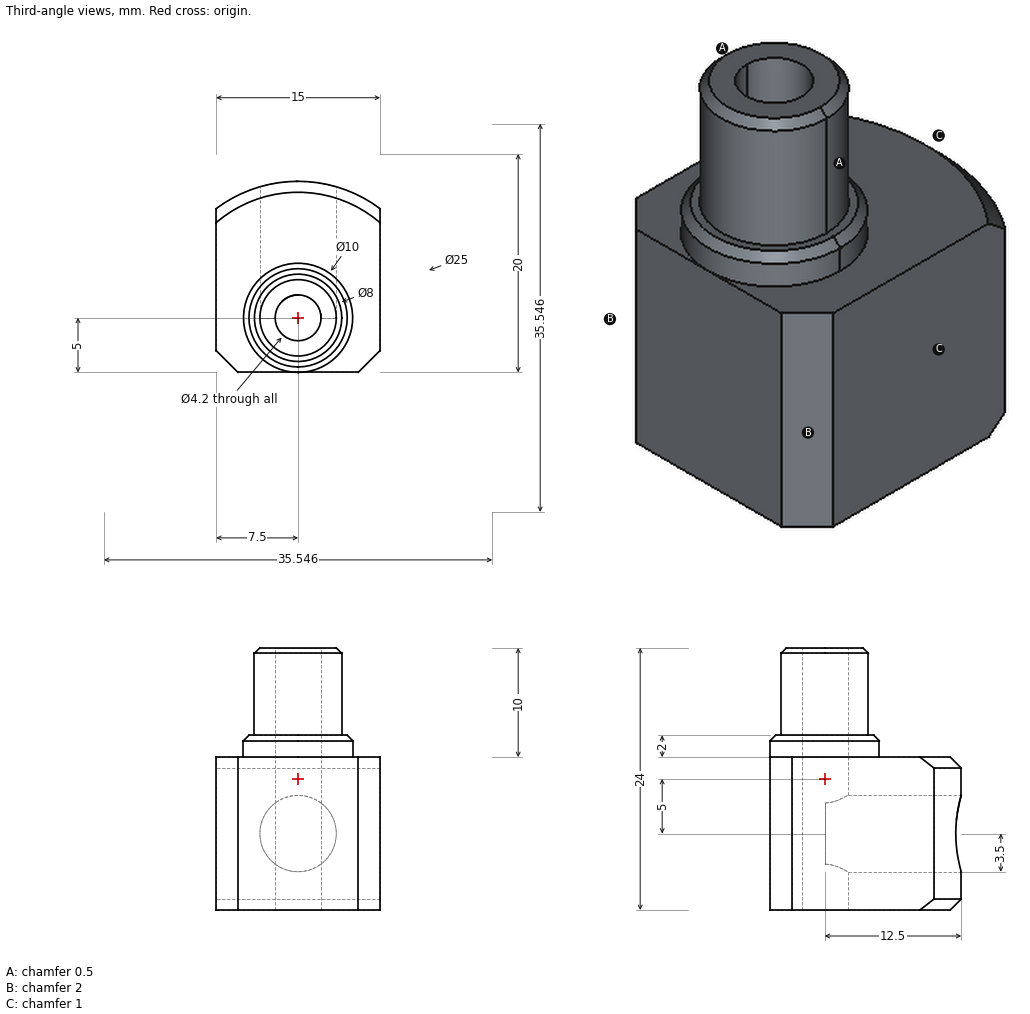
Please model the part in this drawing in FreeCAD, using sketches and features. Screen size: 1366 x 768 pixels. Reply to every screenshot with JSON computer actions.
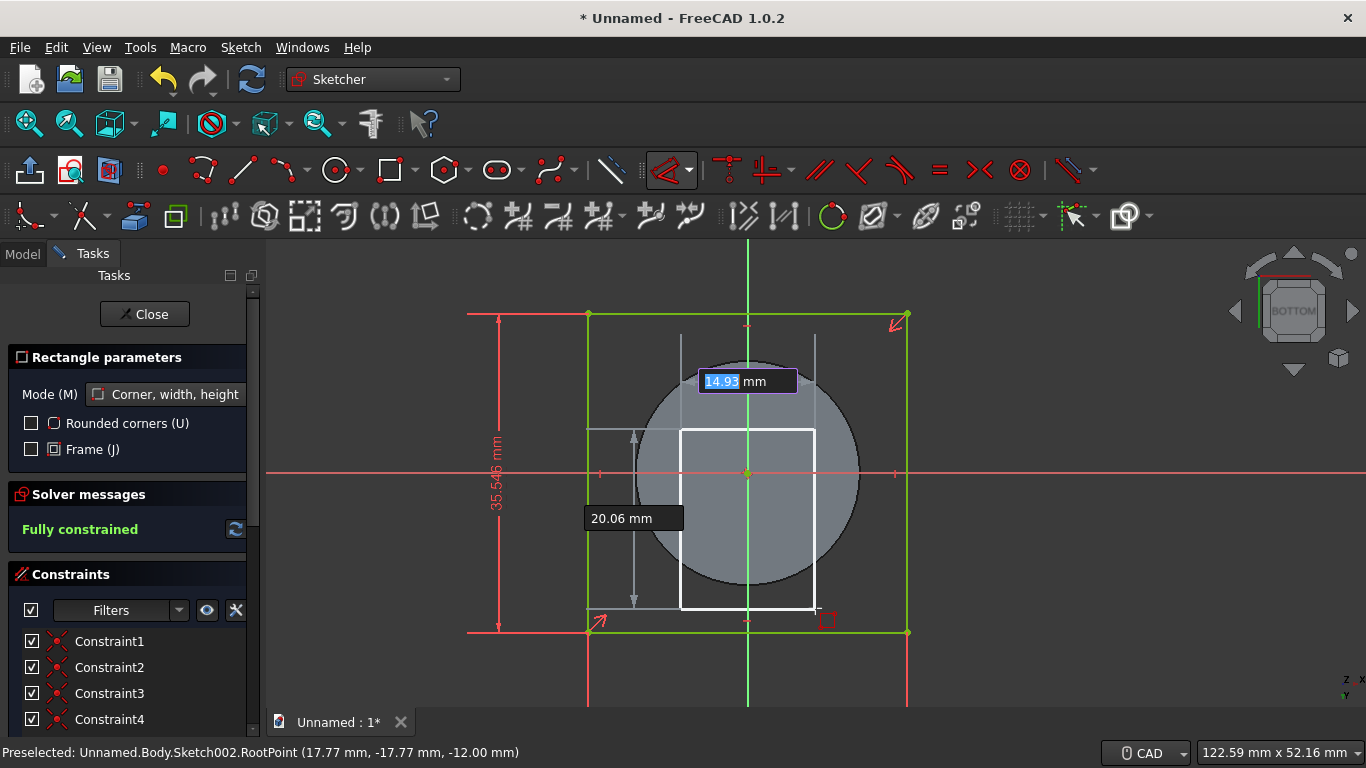
{"action": "type", "text": "15"}
{"action": "key", "text": "Tab"}
{"action": "type", "text": "20"}
{"action": "key", "text": "Return"}
{"action": "key", "text": "Escape"}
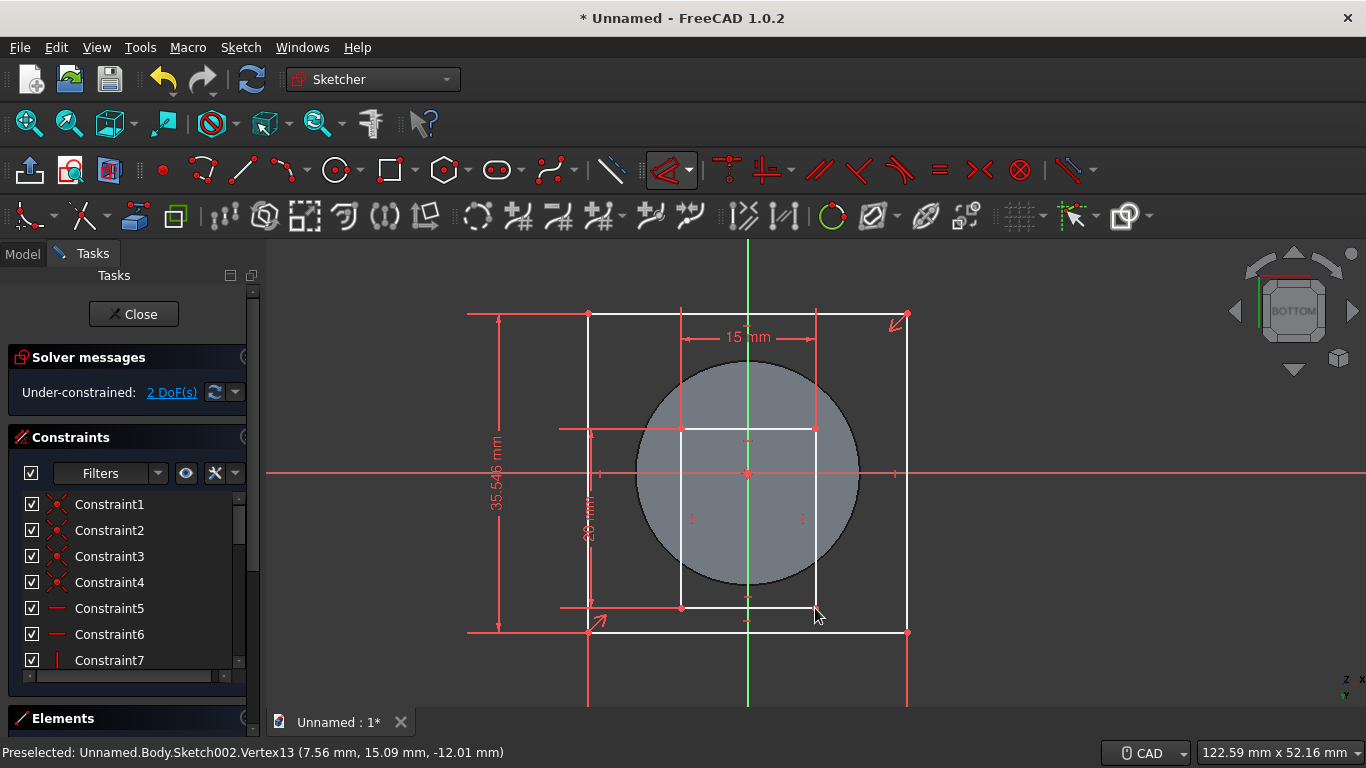
{"action": "left_click", "coordinate": [666, 170]}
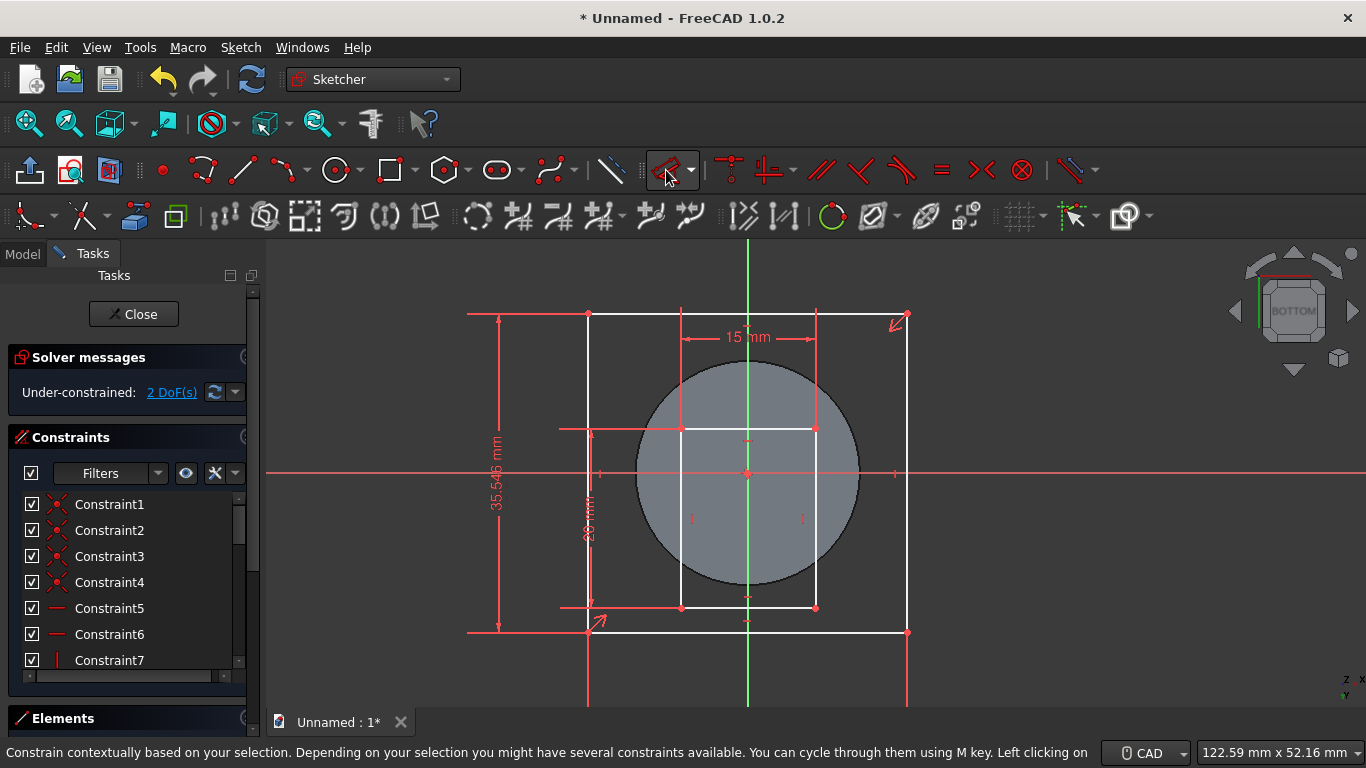
{"action": "left_click", "coordinate": [681, 429]}
{"action": "left_click", "coordinate": [647, 451]}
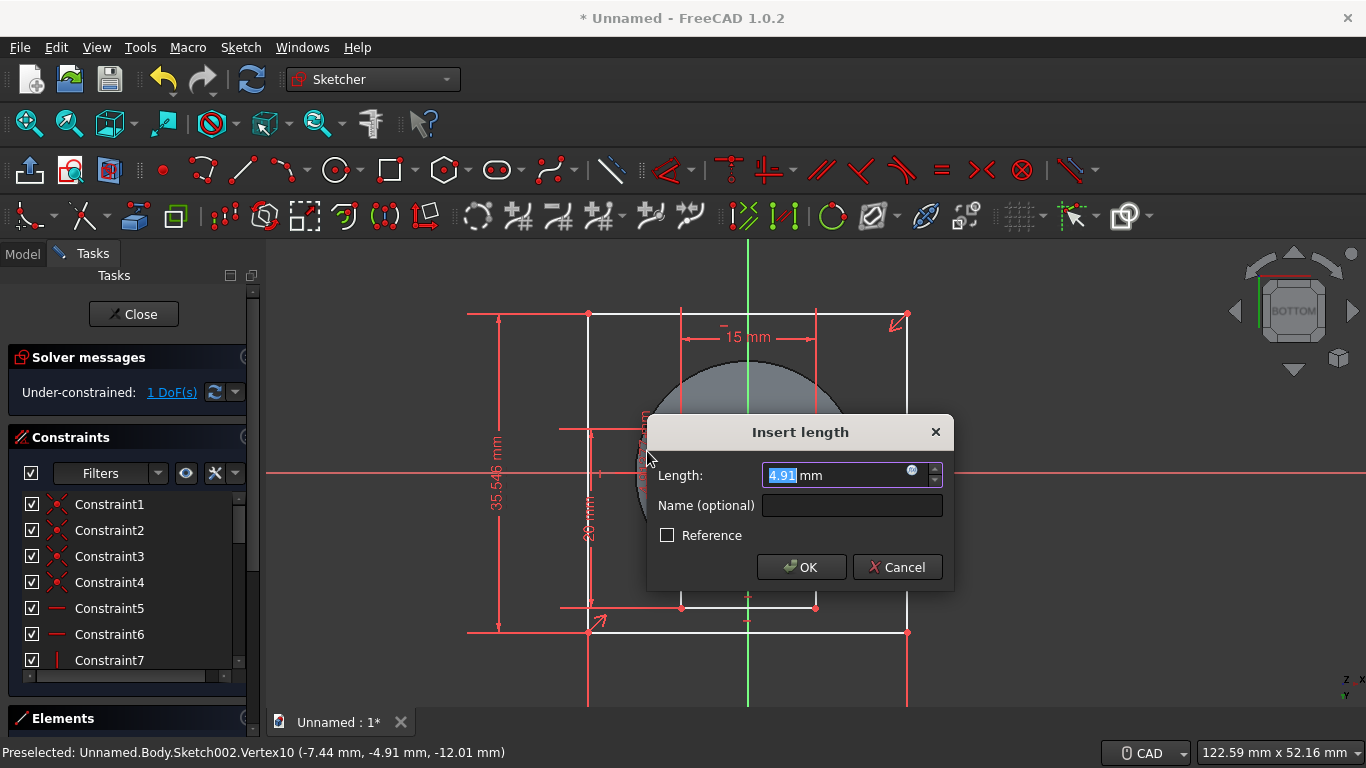
{"action": "type", "text": "5"}
{"action": "key", "text": "Return"}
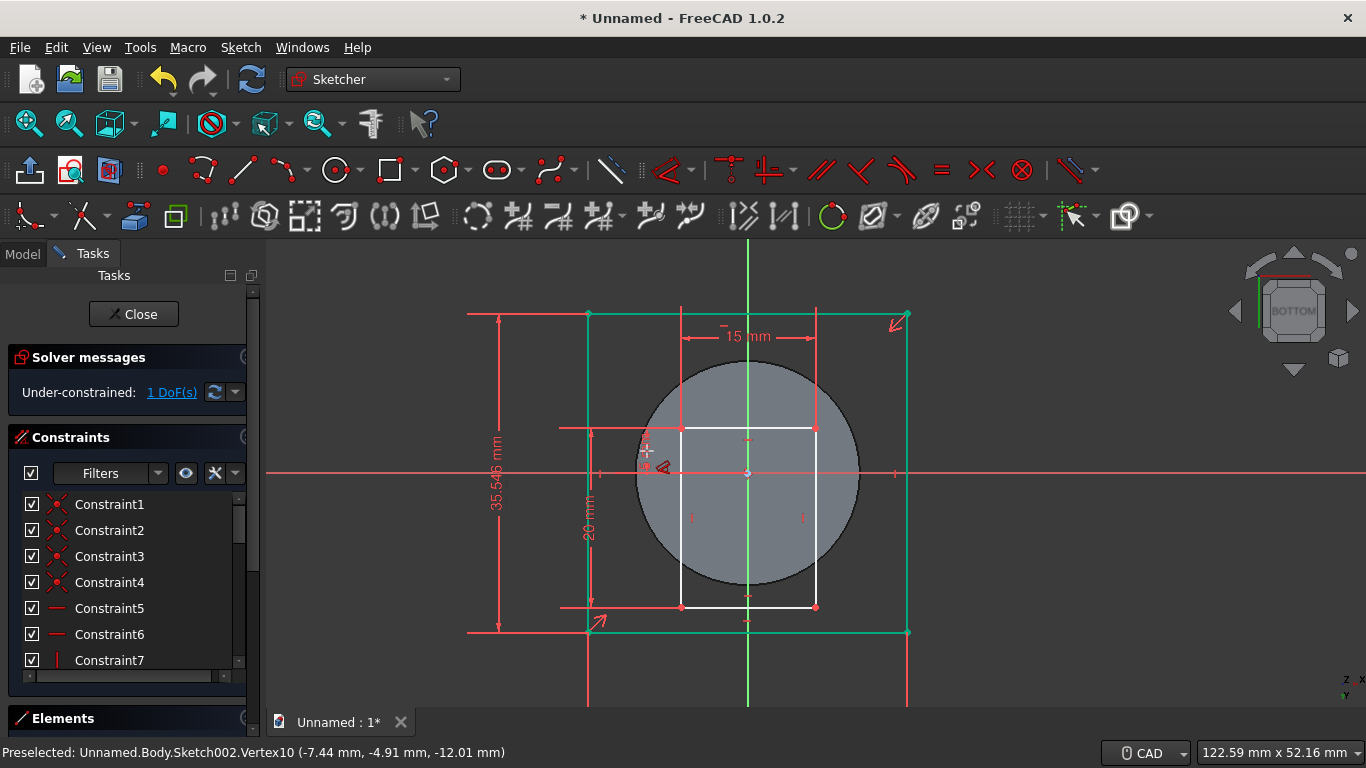
{"action": "left_click", "coordinate": [681, 428]}
{"action": "left_click", "coordinate": [714, 394]}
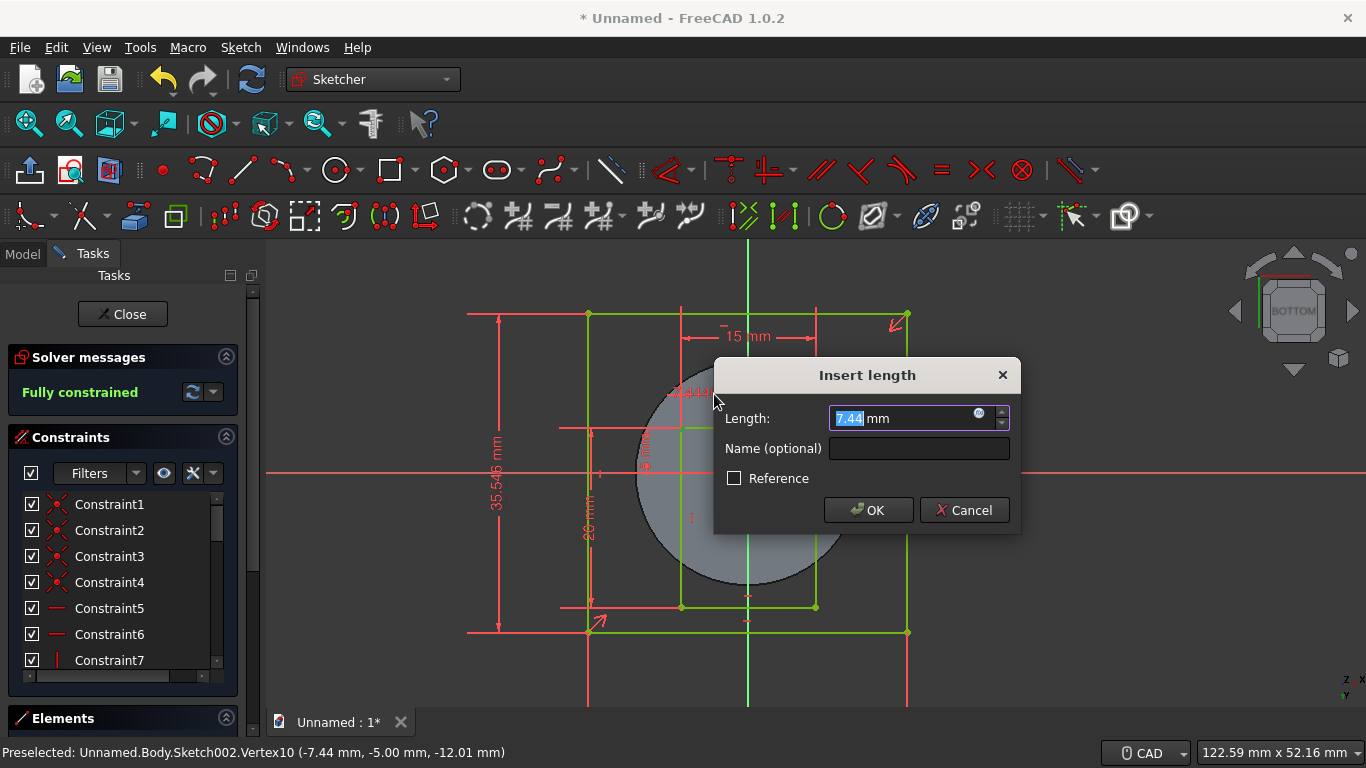
{"action": "type", "text": "7.5"}
{"action": "key", "text": "Return"}
{"action": "key", "text": "Escape"}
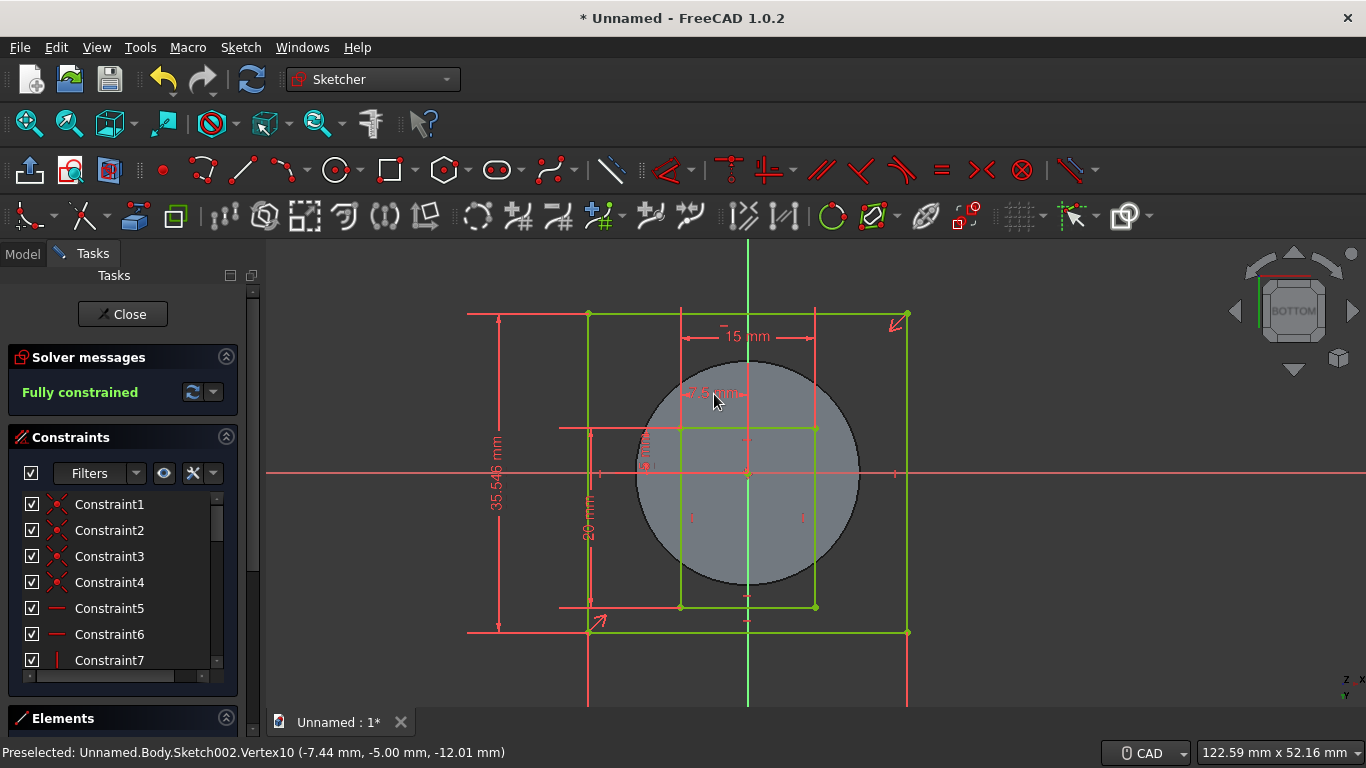
{"action": "left_click", "coordinate": [123, 314]}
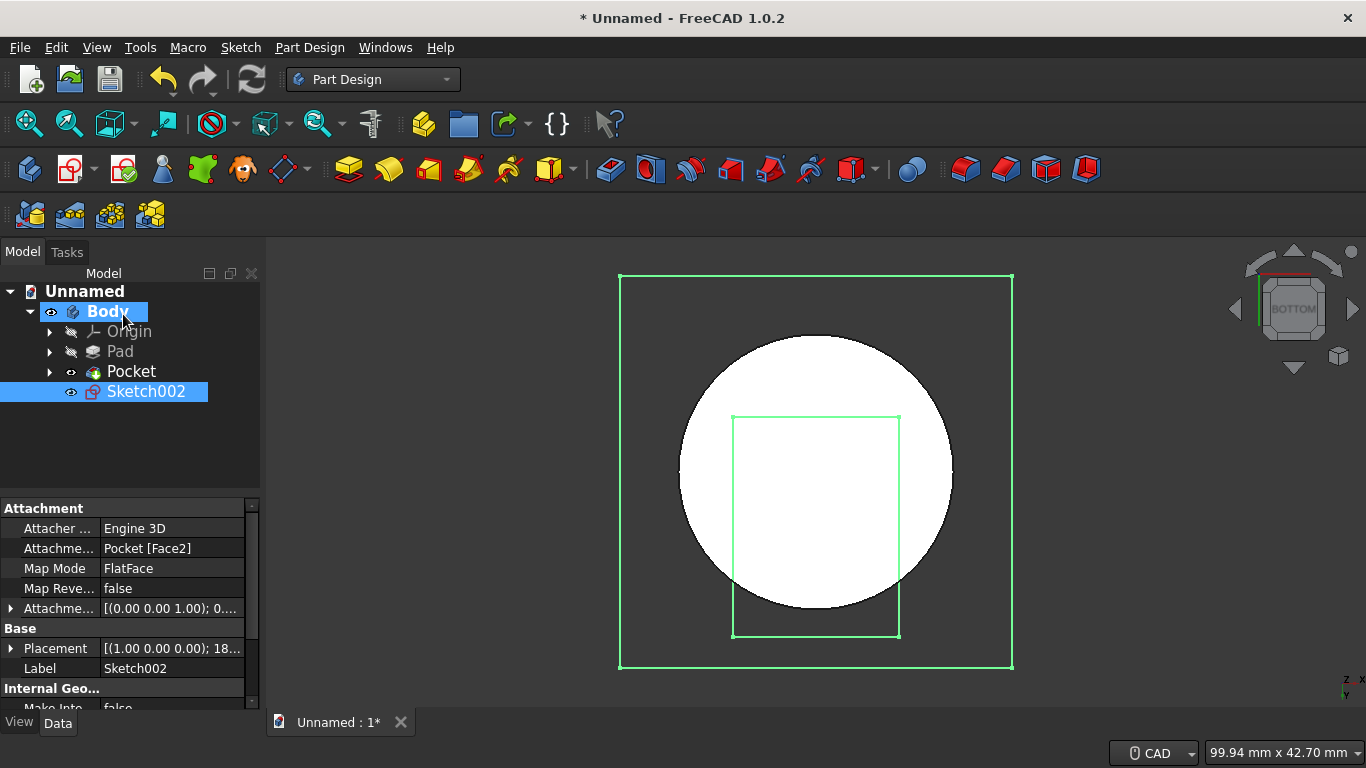
{"action": "left_click", "coordinate": [612, 170]}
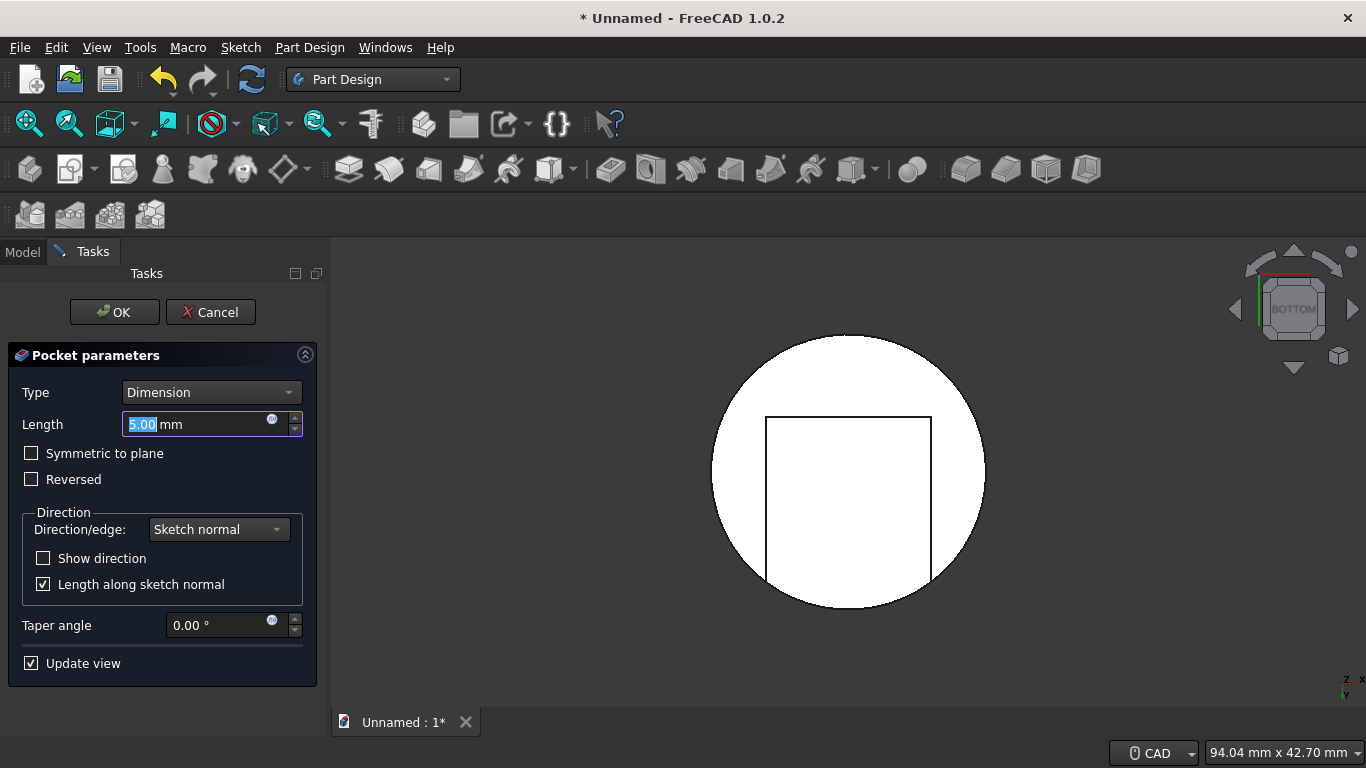
{"action": "left_click", "coordinate": [212, 392]}